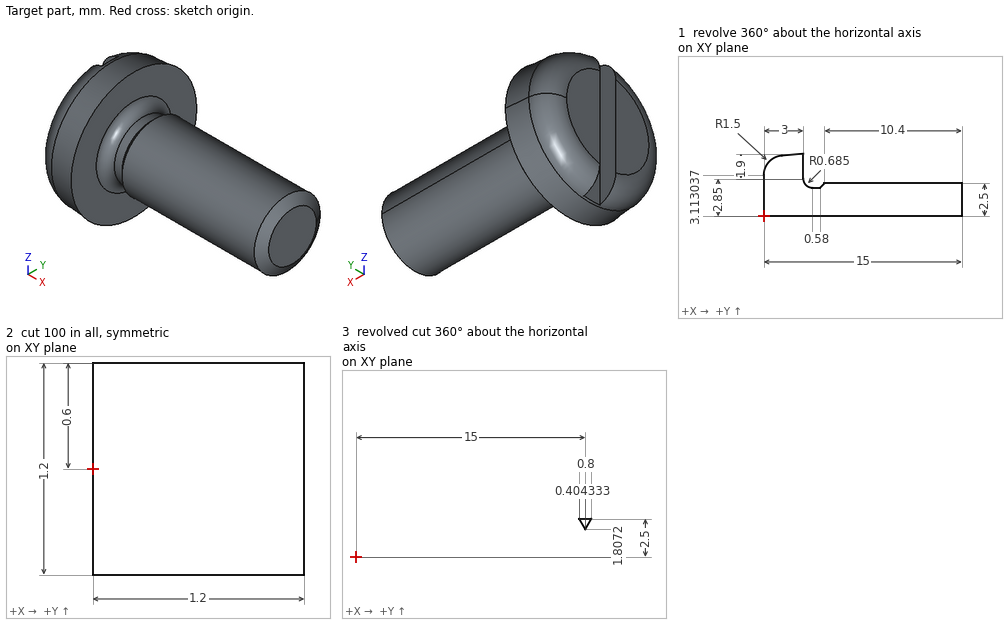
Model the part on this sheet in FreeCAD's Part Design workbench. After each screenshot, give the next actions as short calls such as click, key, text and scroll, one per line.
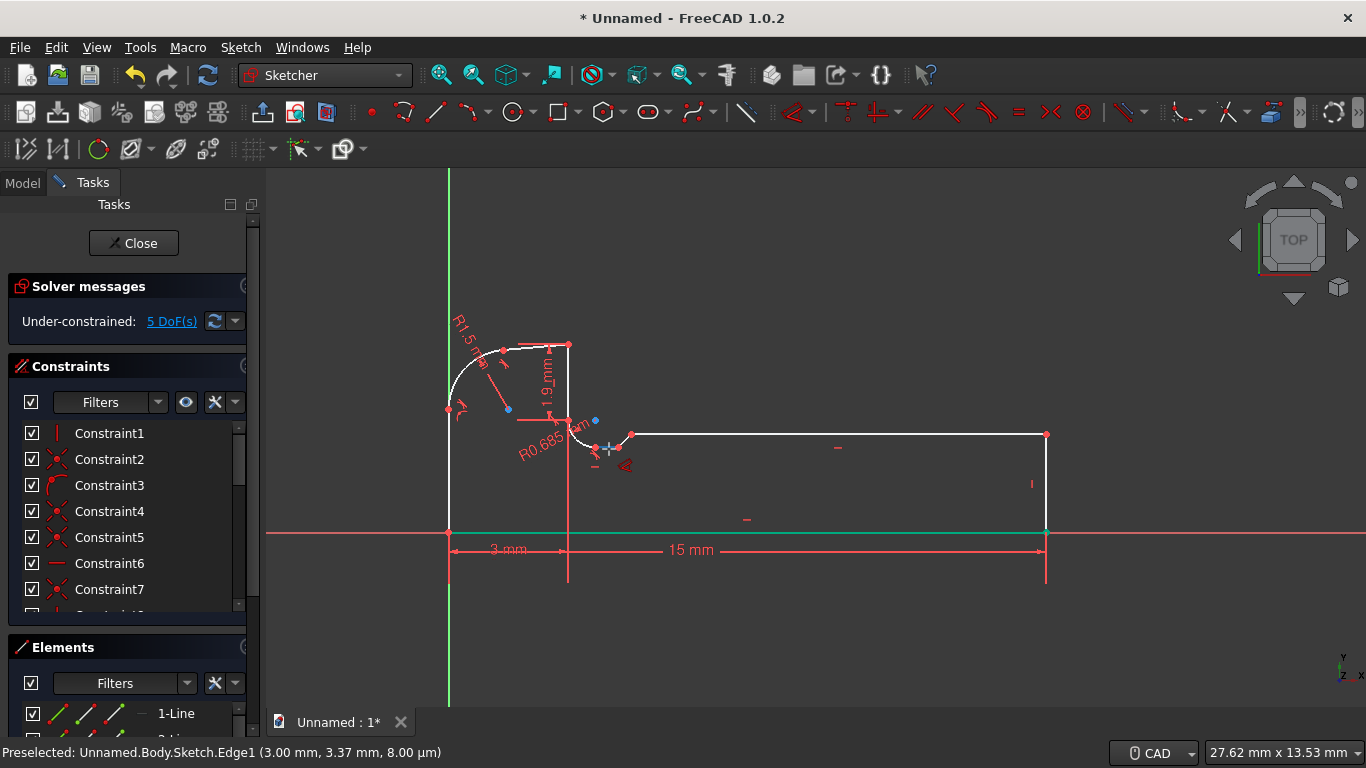
click(1046, 503)
click(1080, 483)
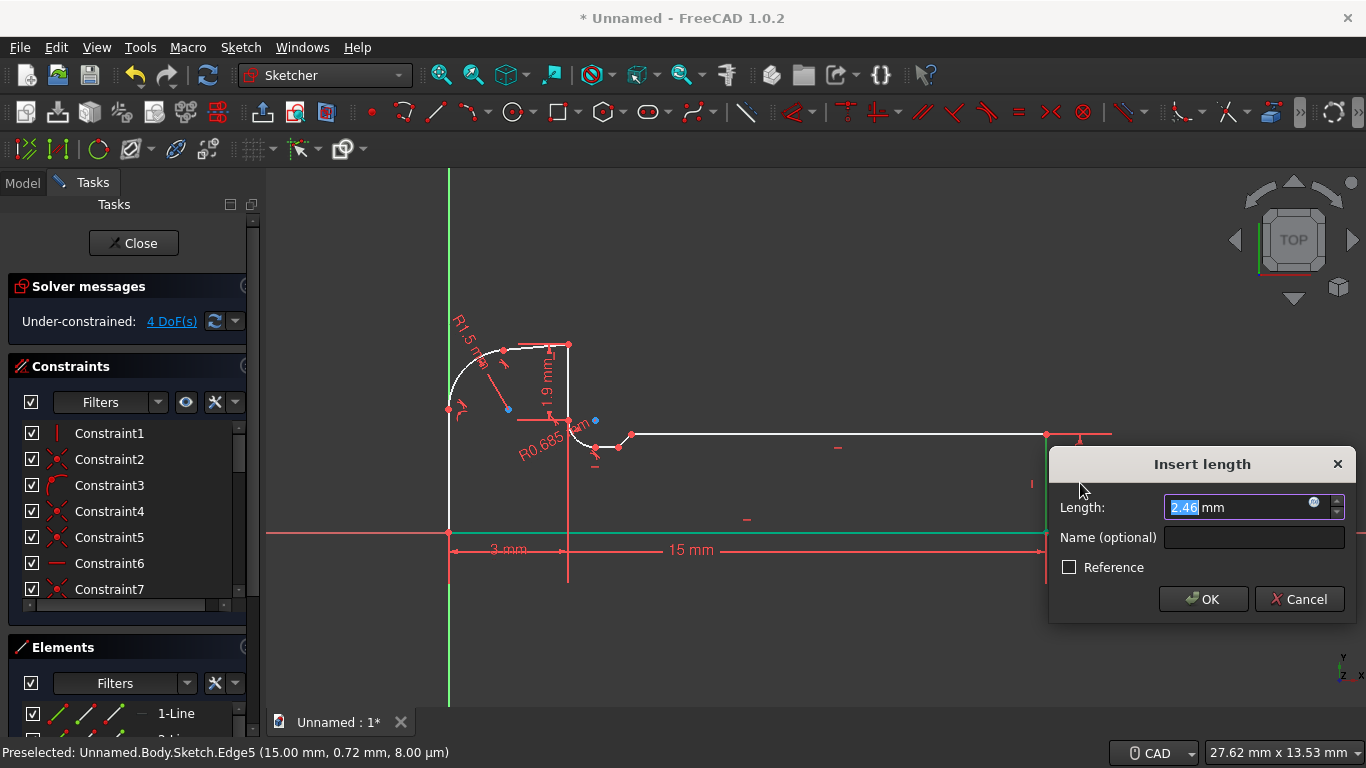
text(2.5)
key(Return)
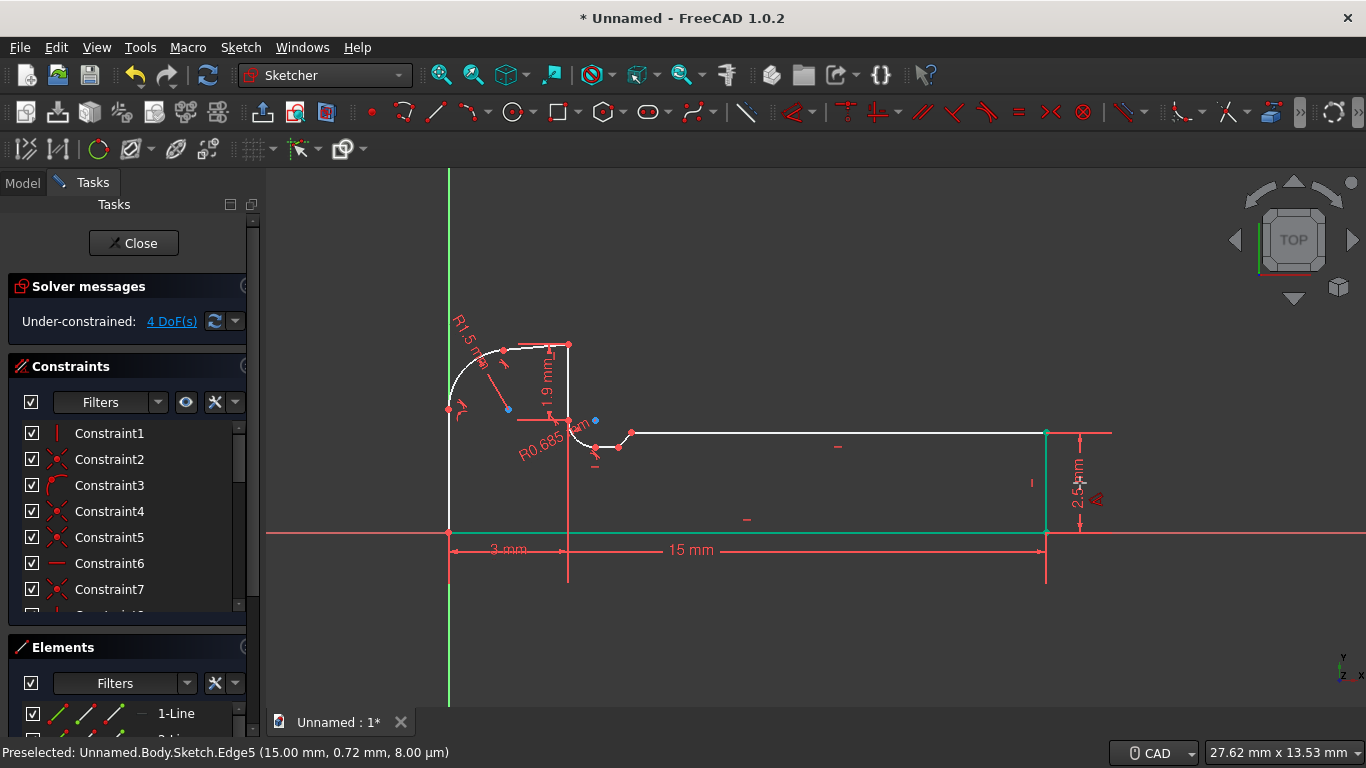
click(922, 433)
click(839, 399)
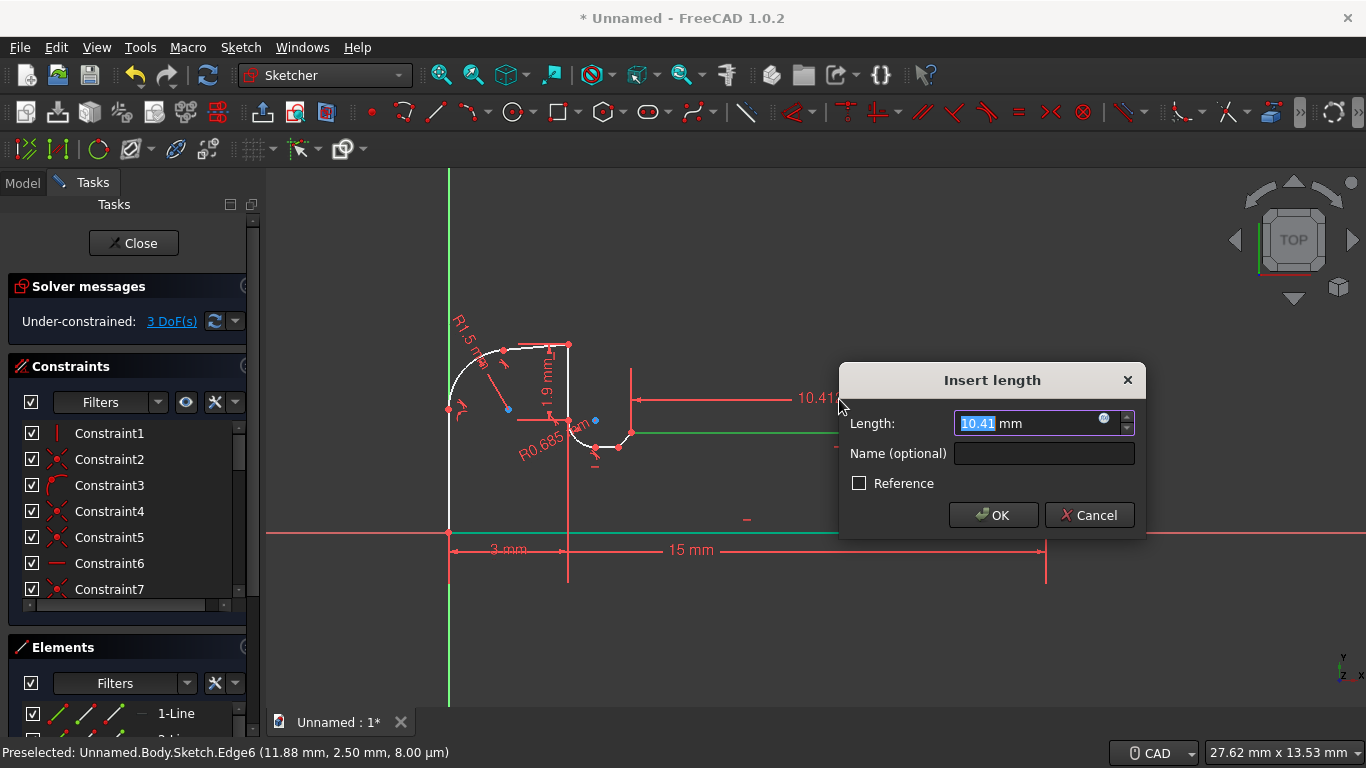
text(10.4)
key(Return)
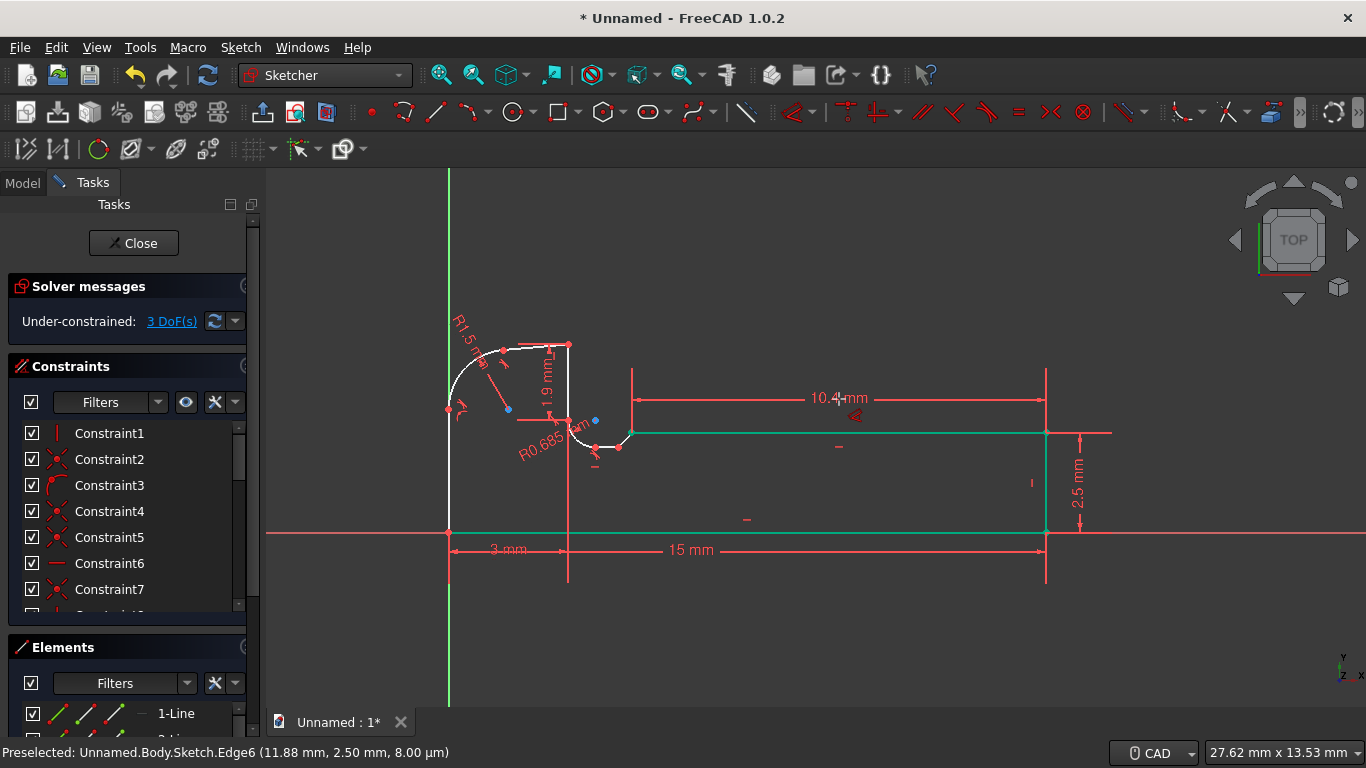
scroll(609, 447, up, 3)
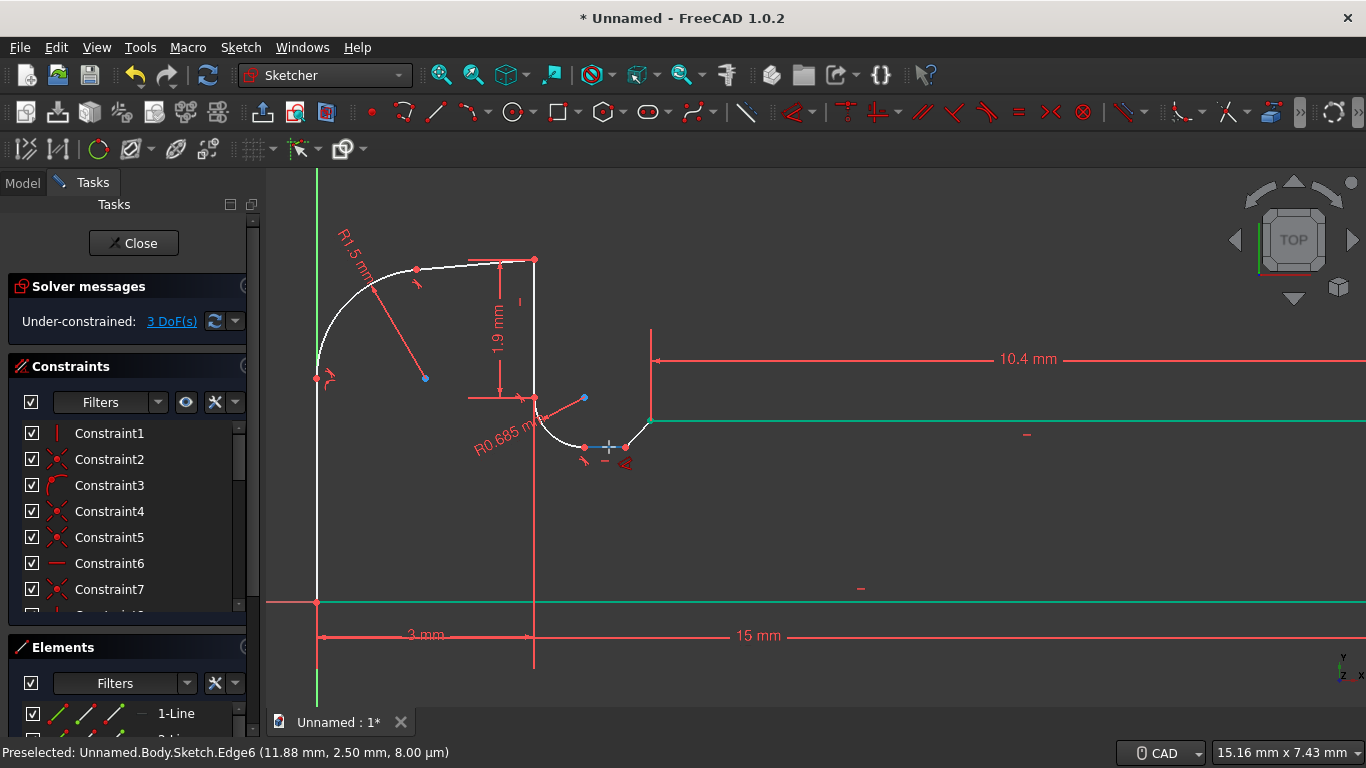
click(609, 447)
click(605, 481)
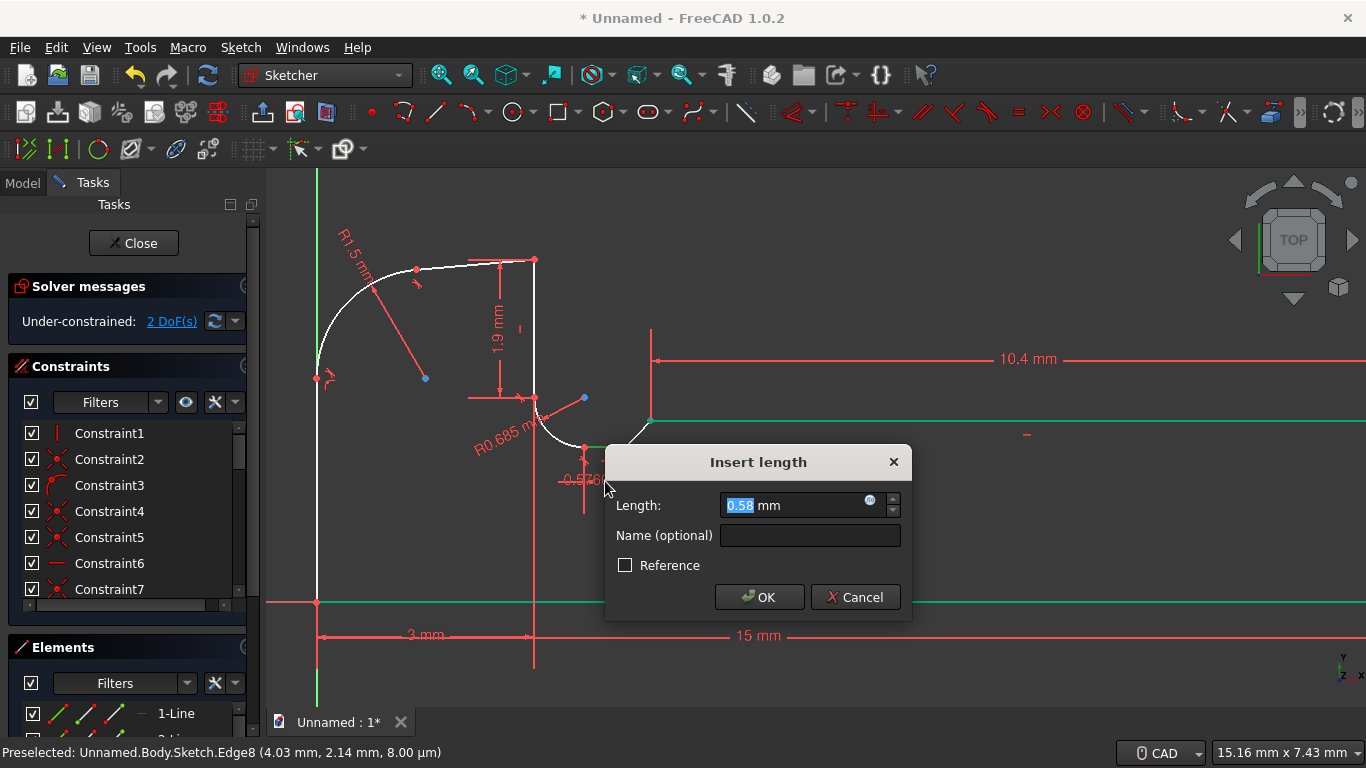
text(0.58)
key(Return)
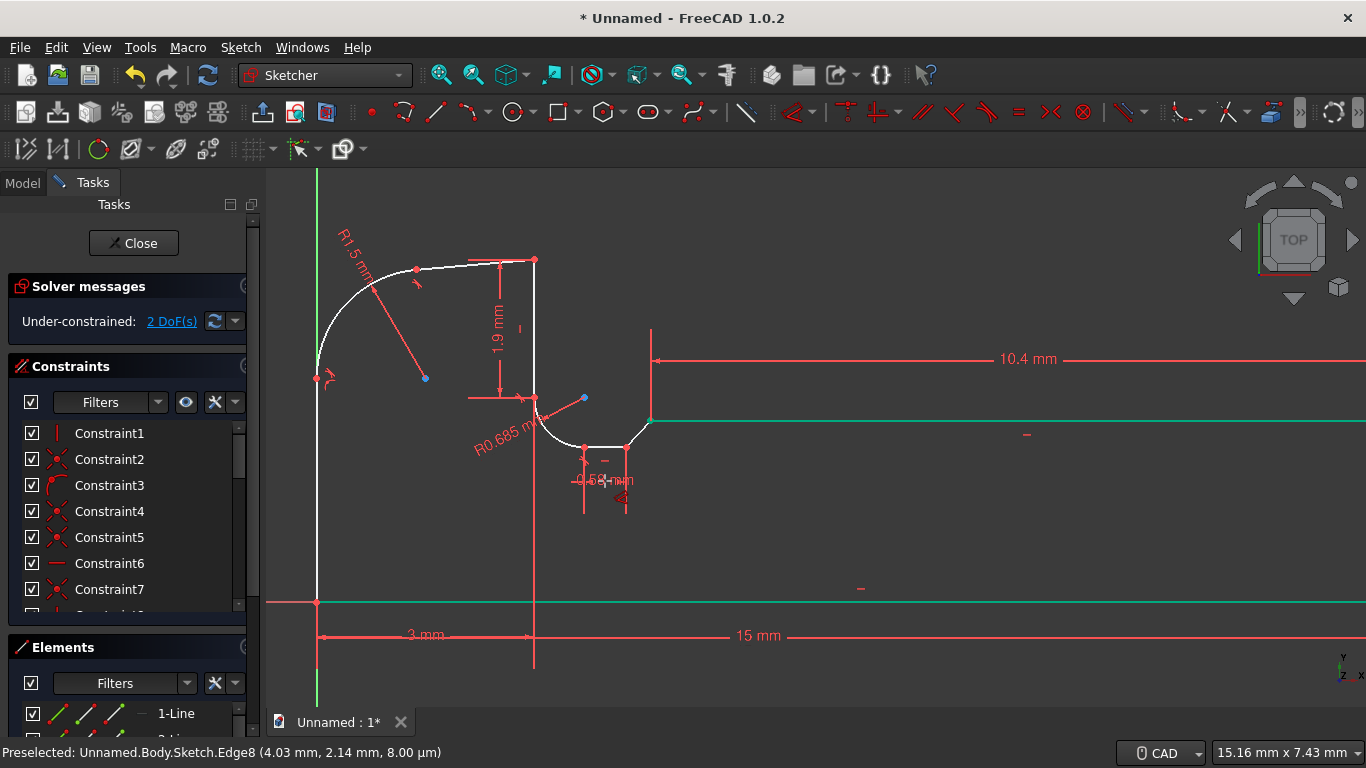
click(534, 398)
click(568, 547)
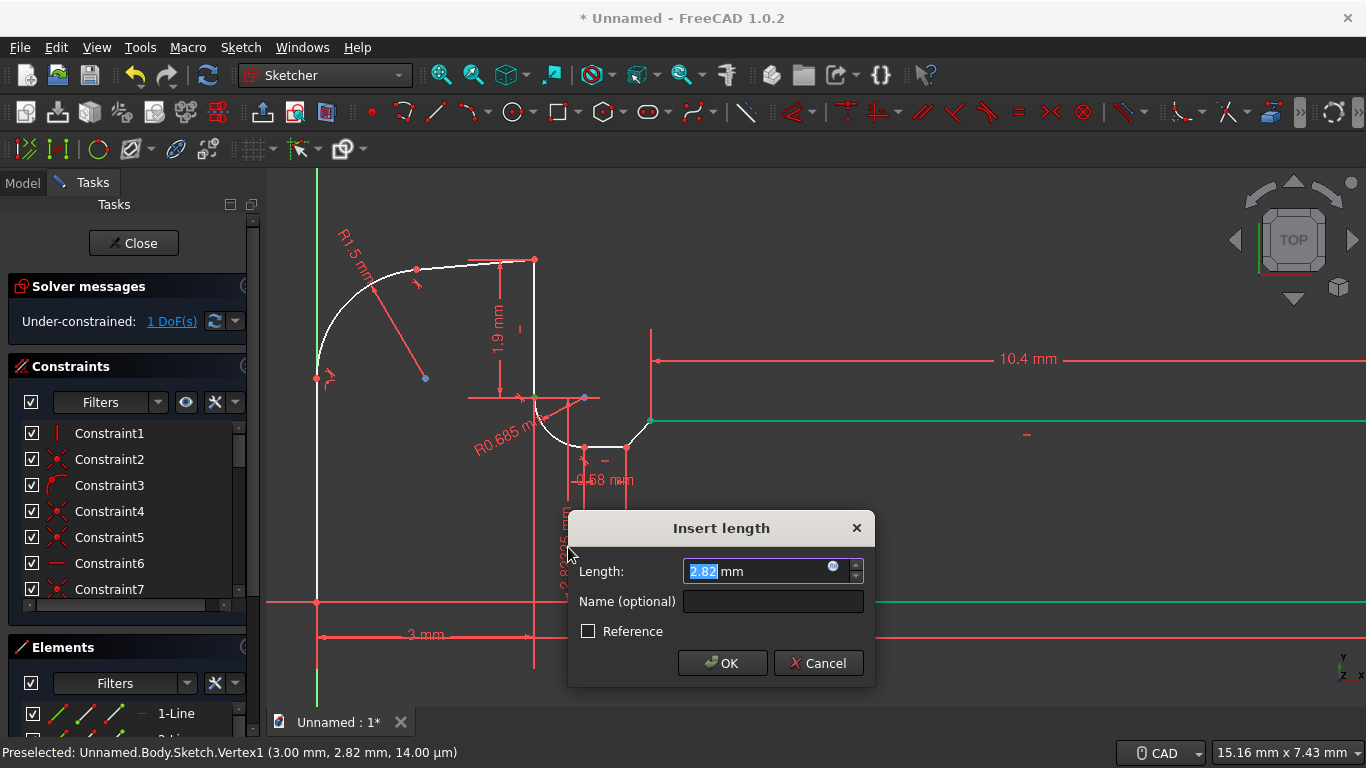
text(2.85)
key(Return)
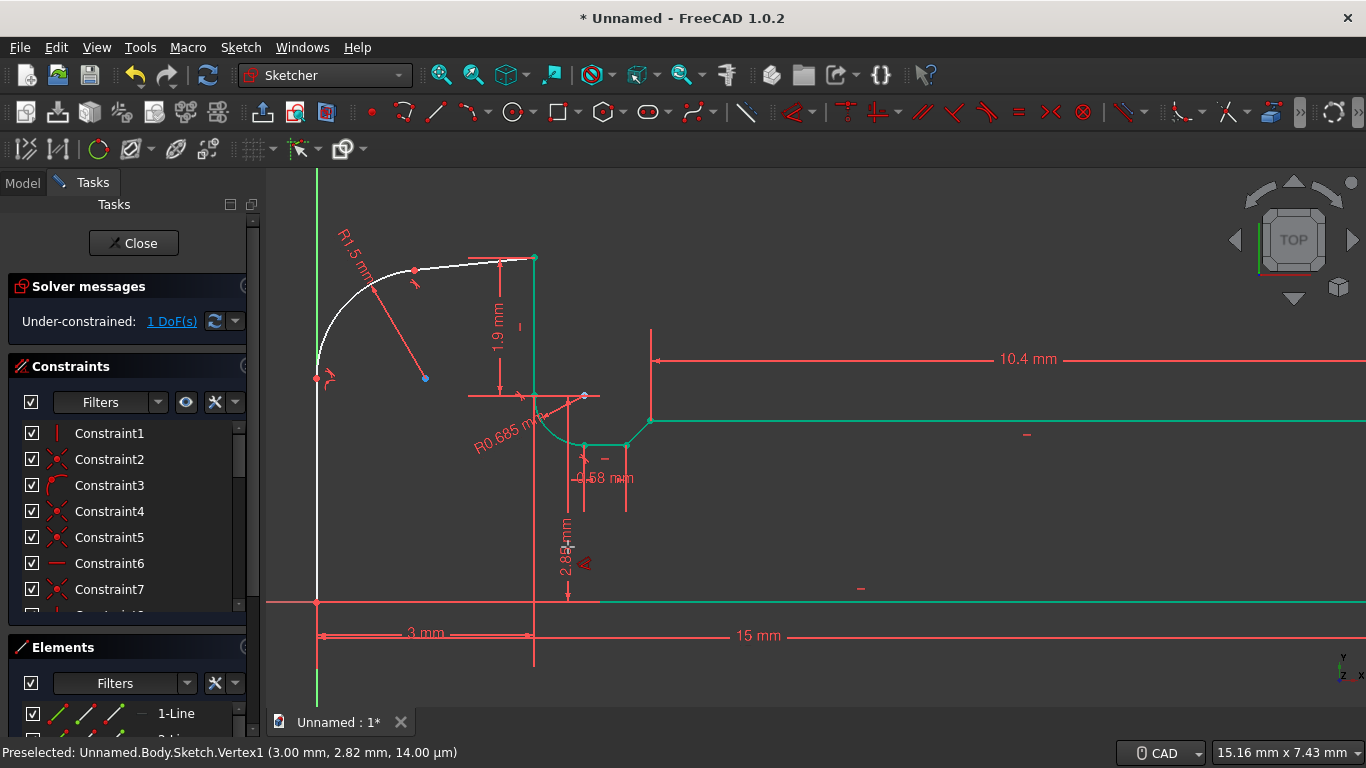
click(317, 446)
click(351, 490)